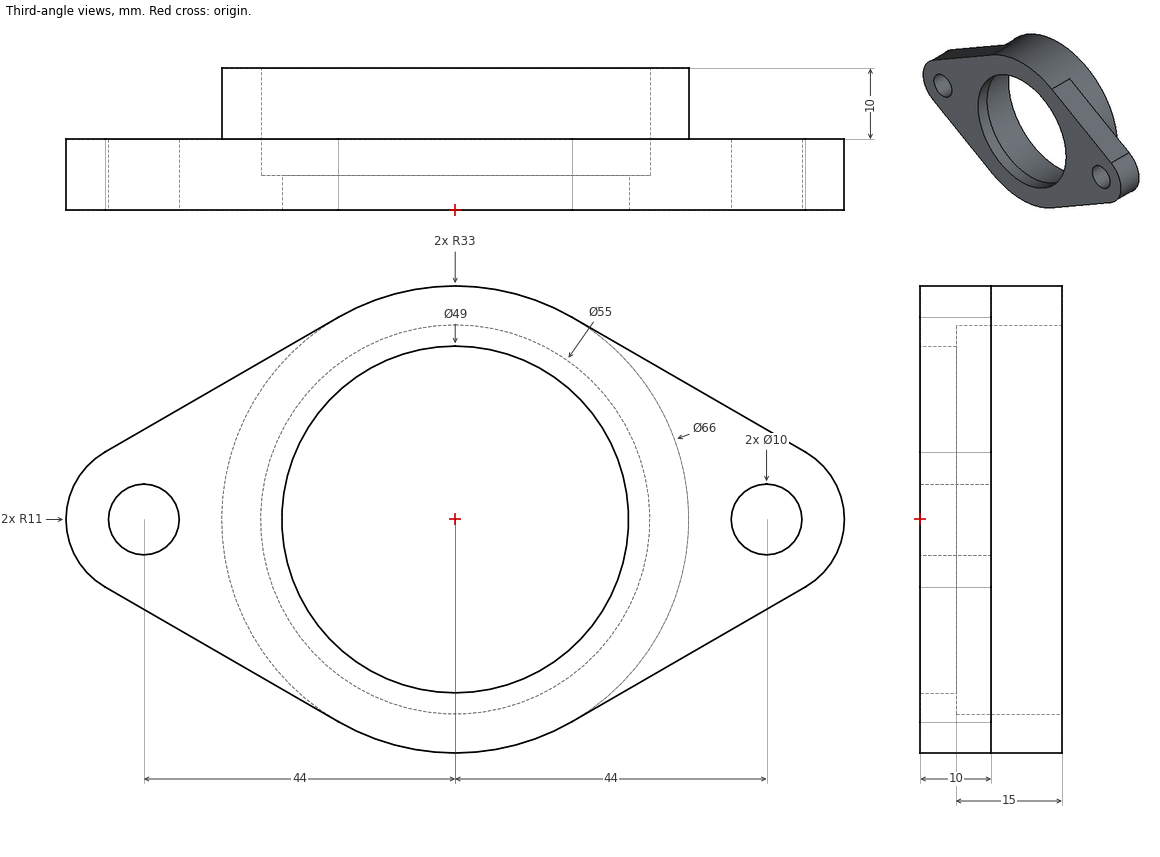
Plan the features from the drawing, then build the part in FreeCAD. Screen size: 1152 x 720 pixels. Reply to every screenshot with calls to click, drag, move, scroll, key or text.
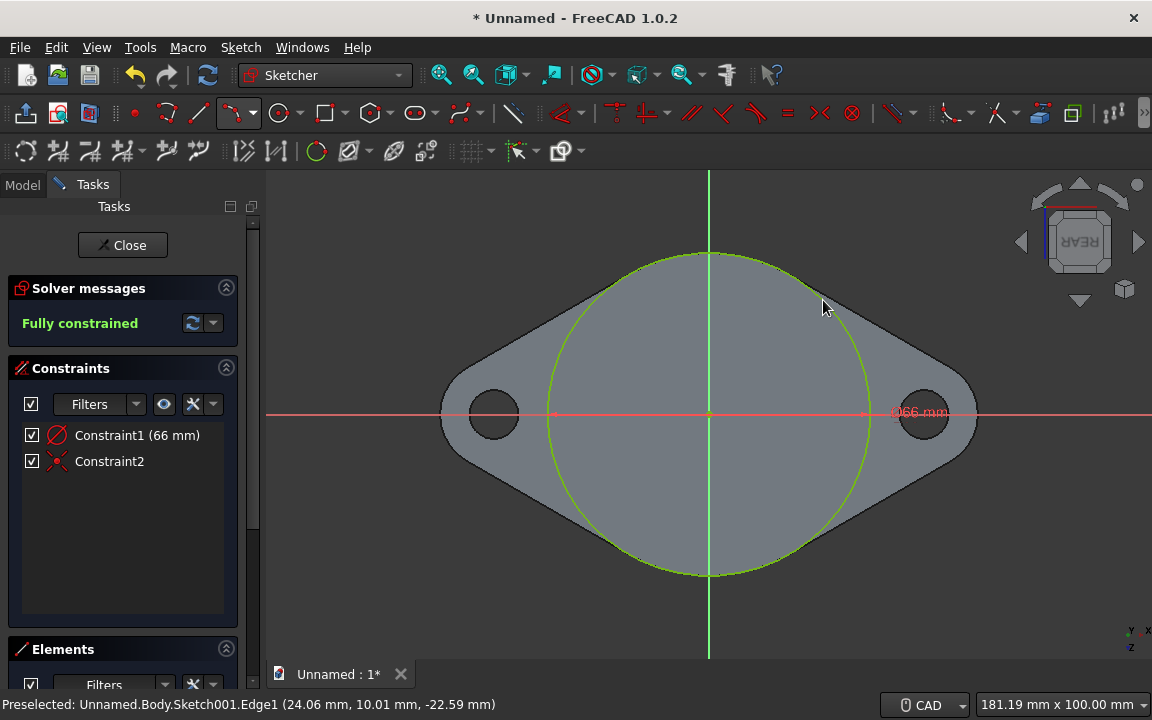
click(123, 245)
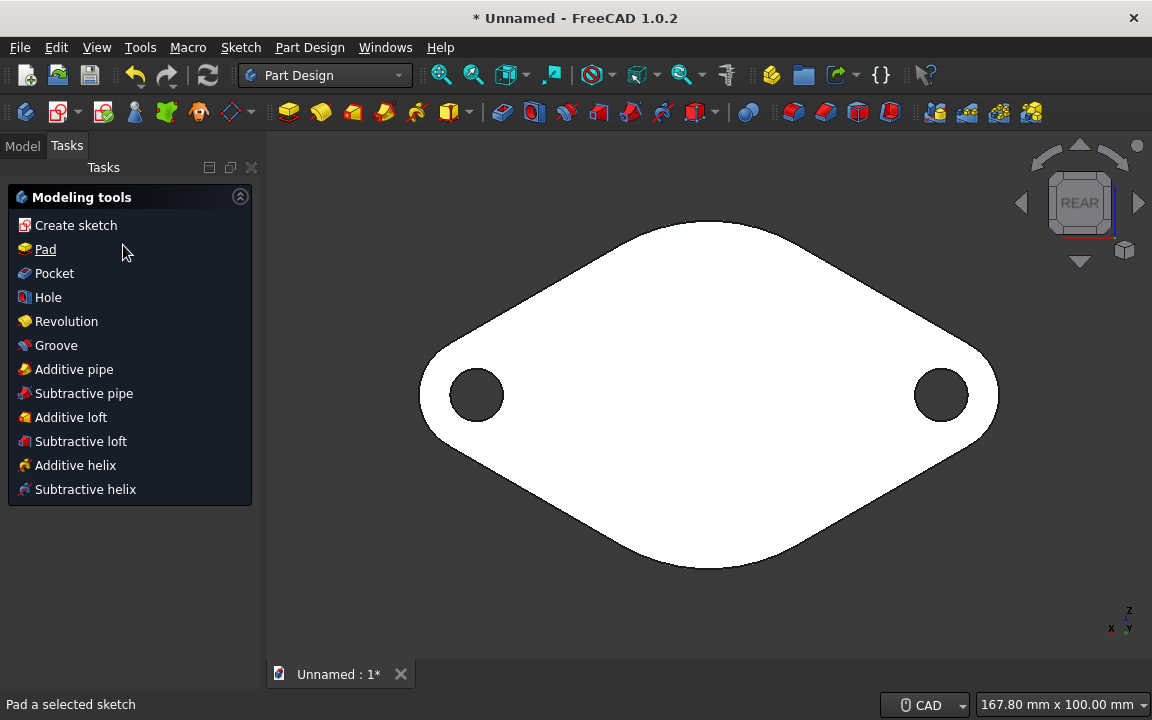
click(290, 112)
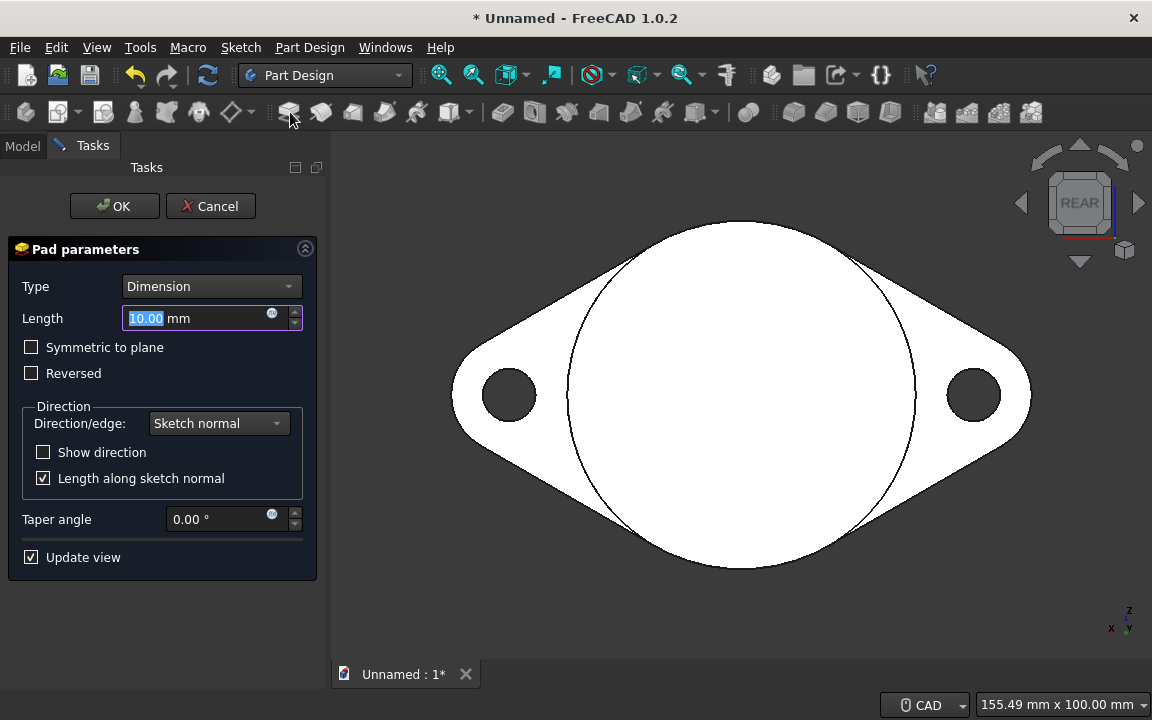
text(10)
key(Tab)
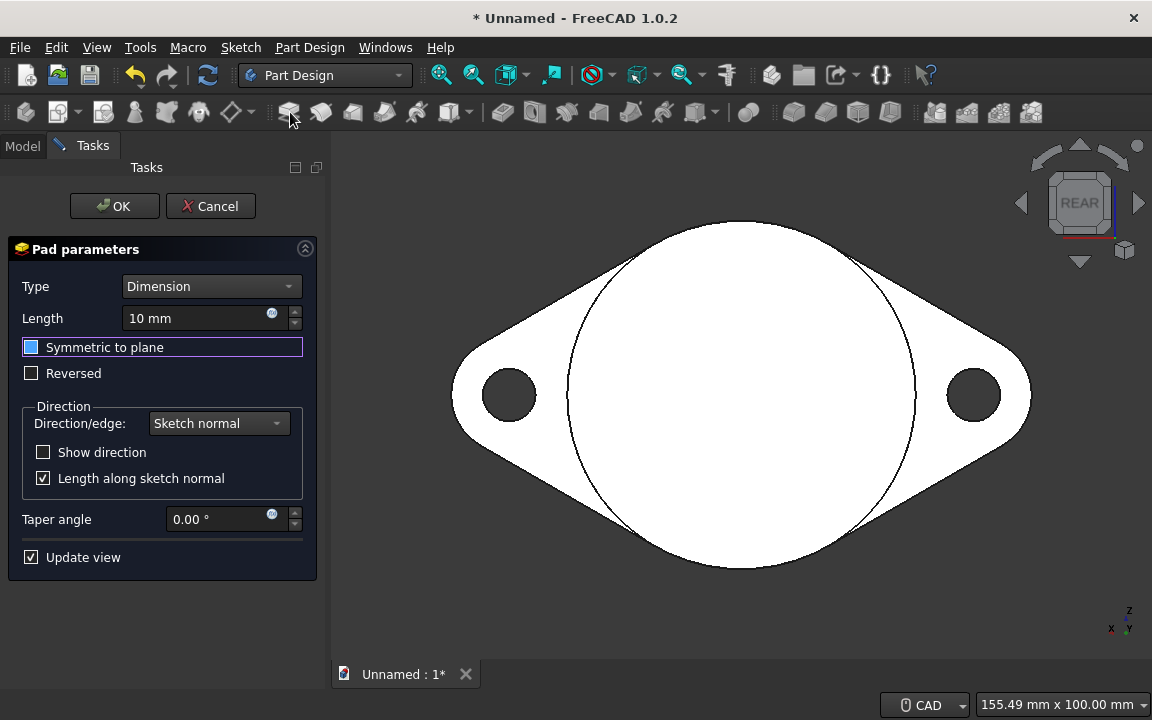
click(115, 206)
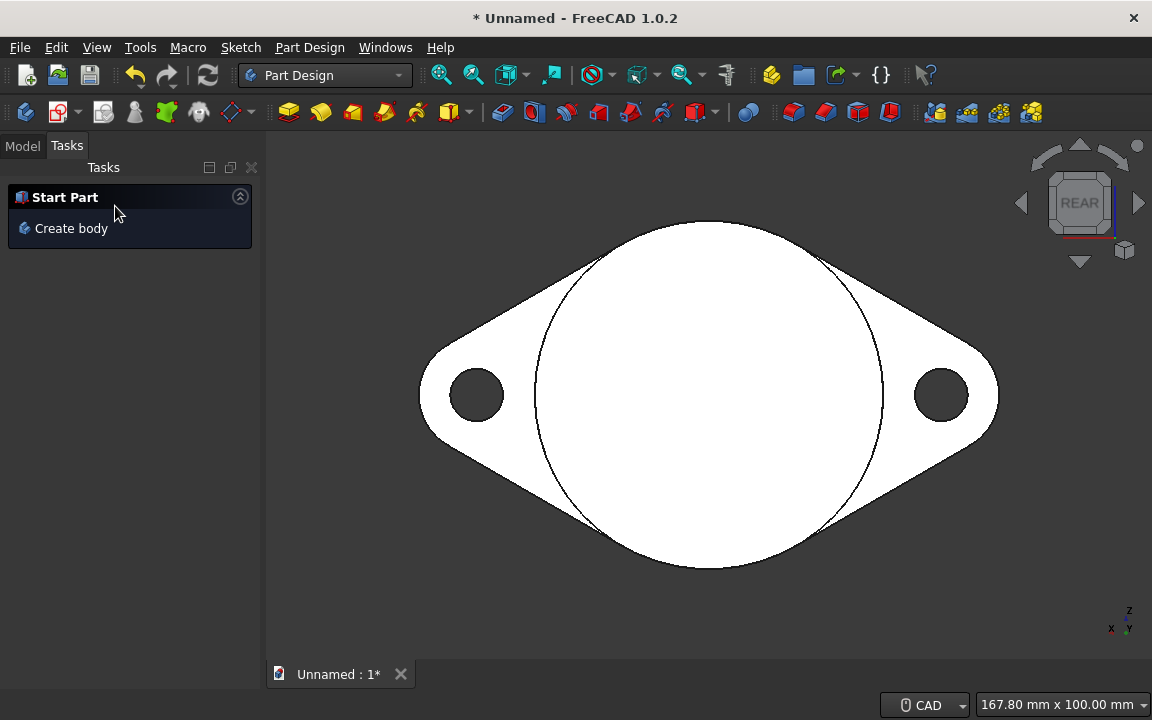
click(709, 394)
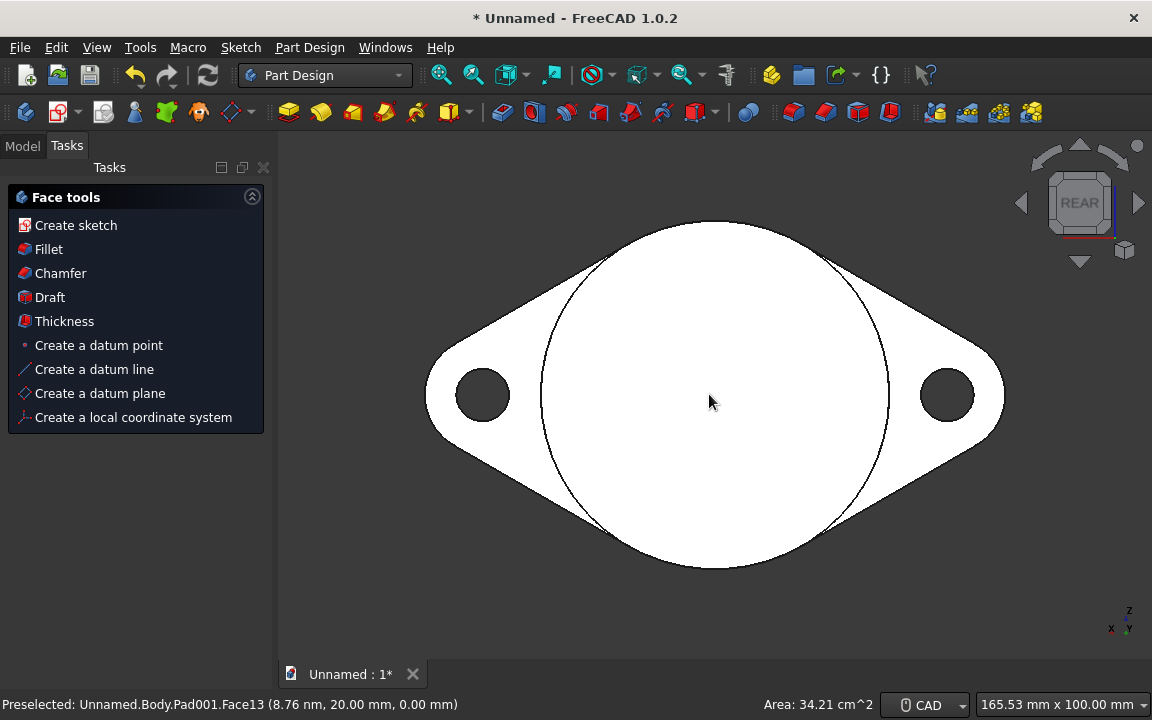
click(58, 112)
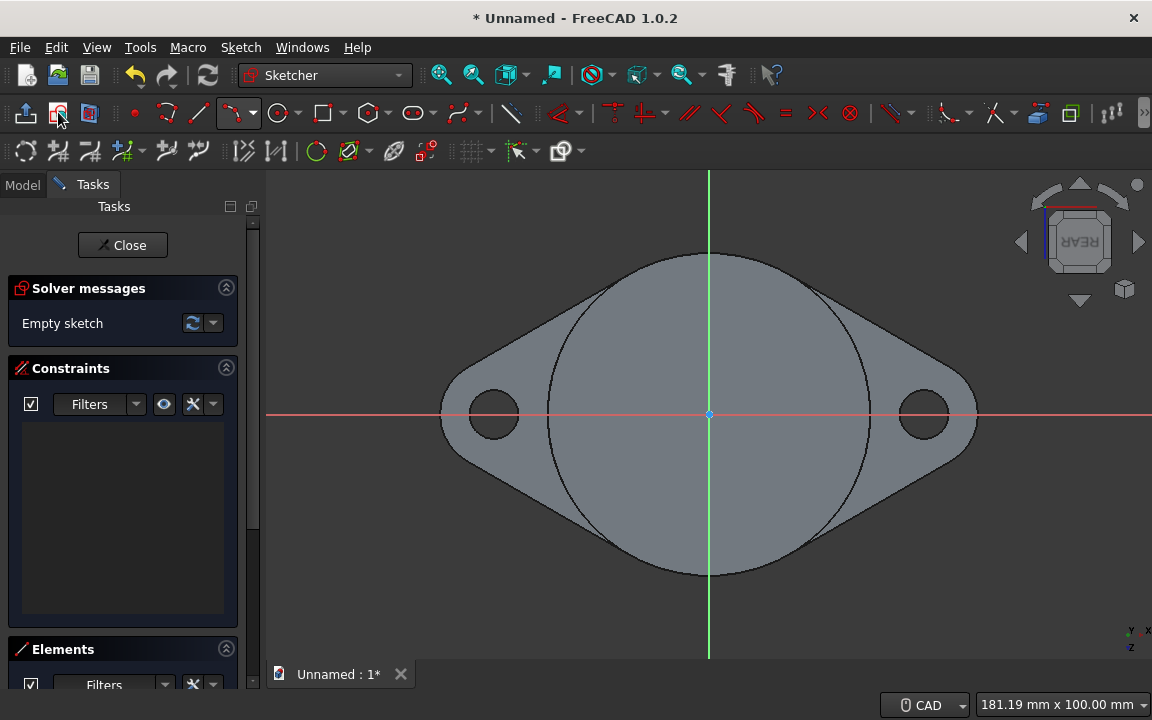
click(278, 114)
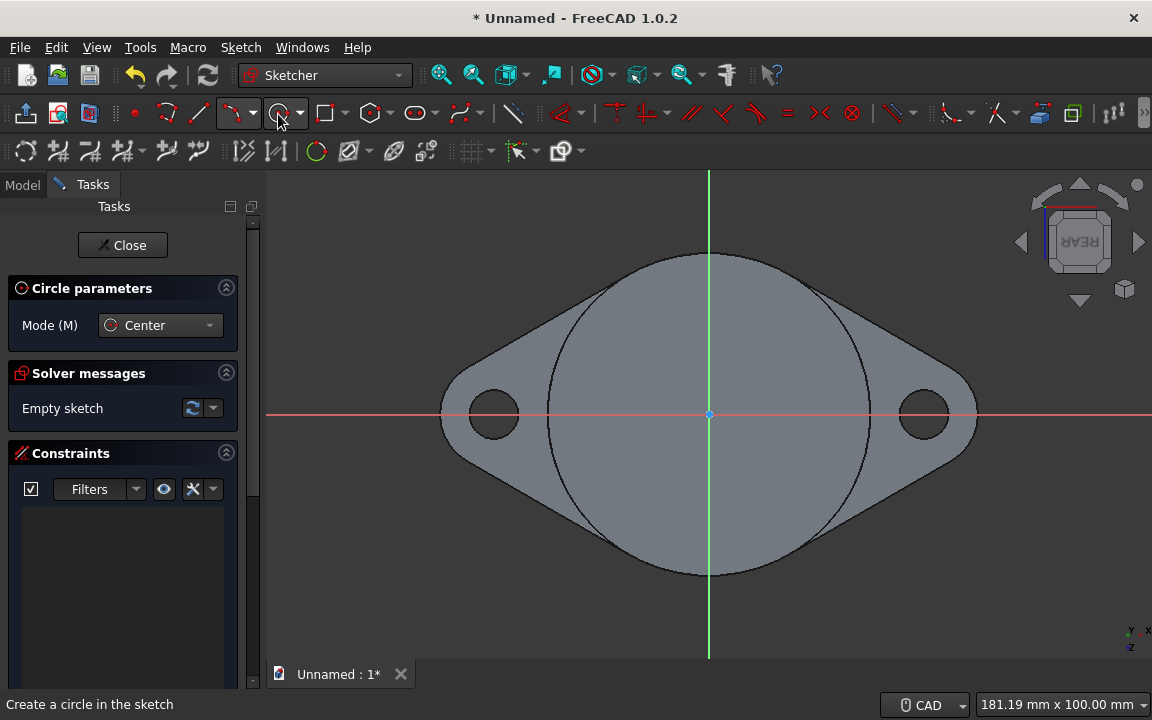
click(709, 414)
move(804, 319)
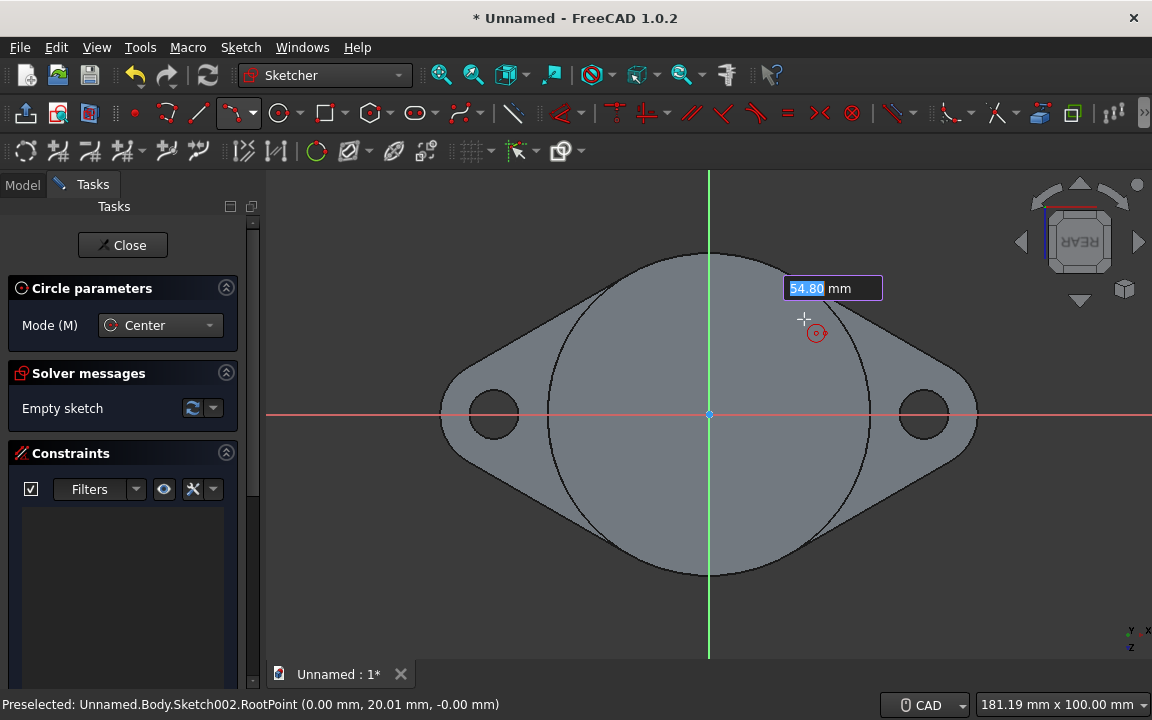
text(55)
key(Return)
key(Escape)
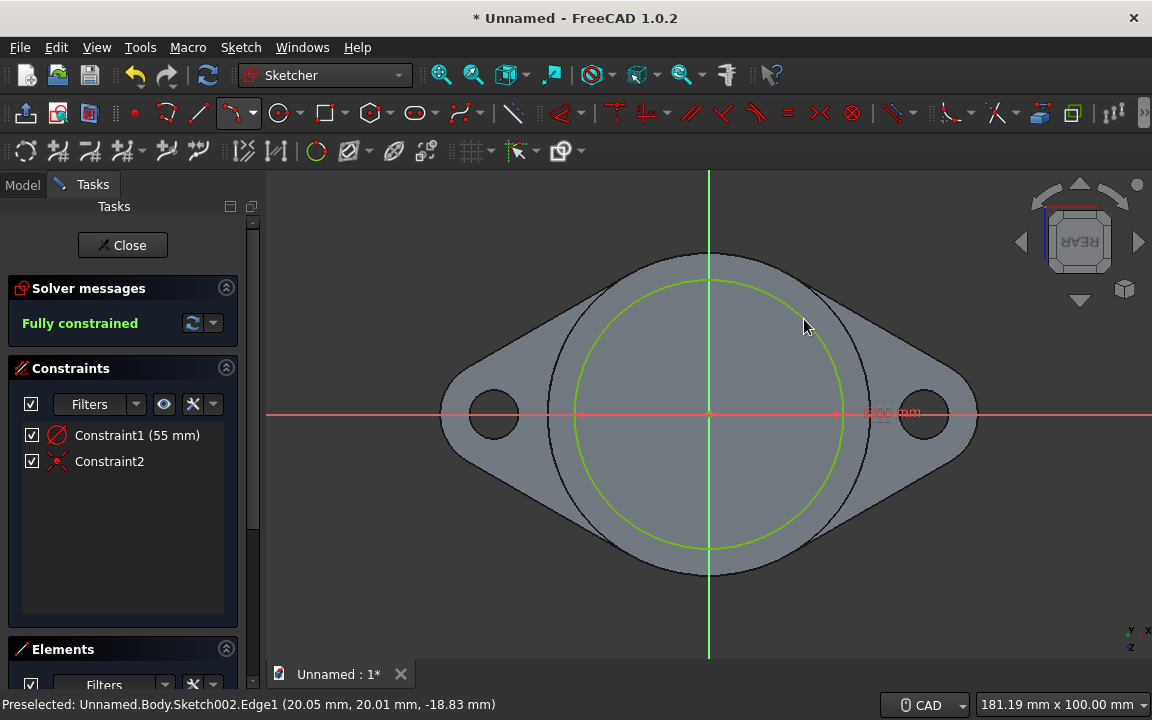
click(123, 245)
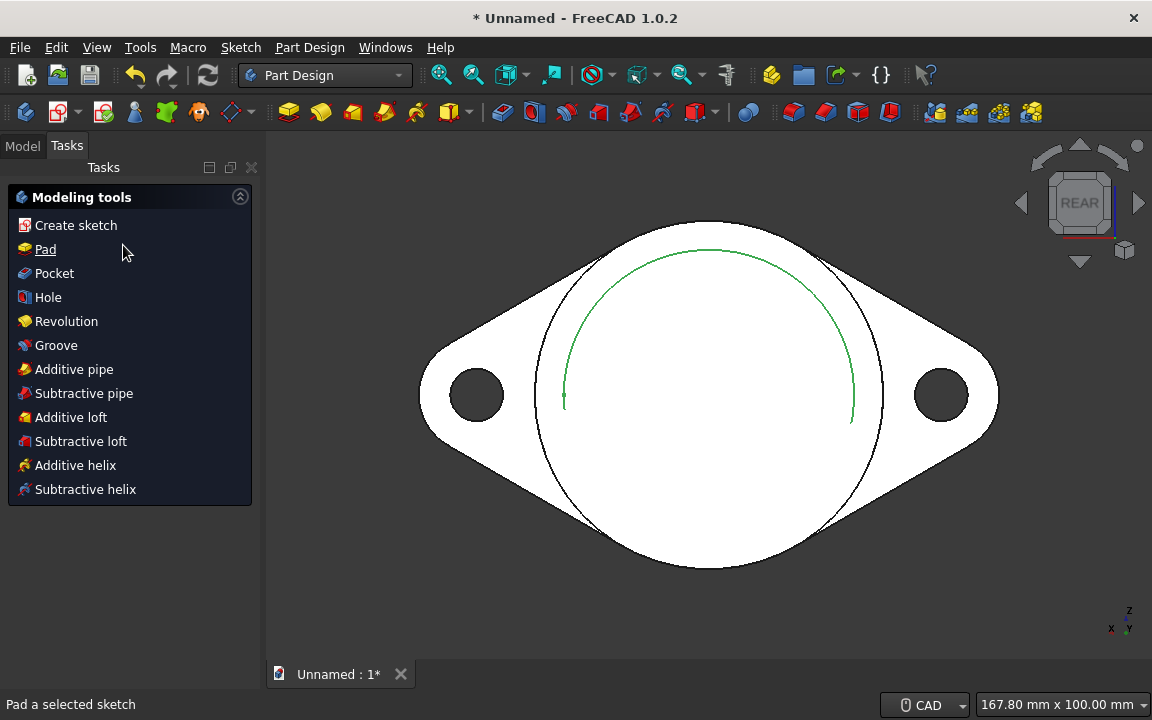
click(504, 112)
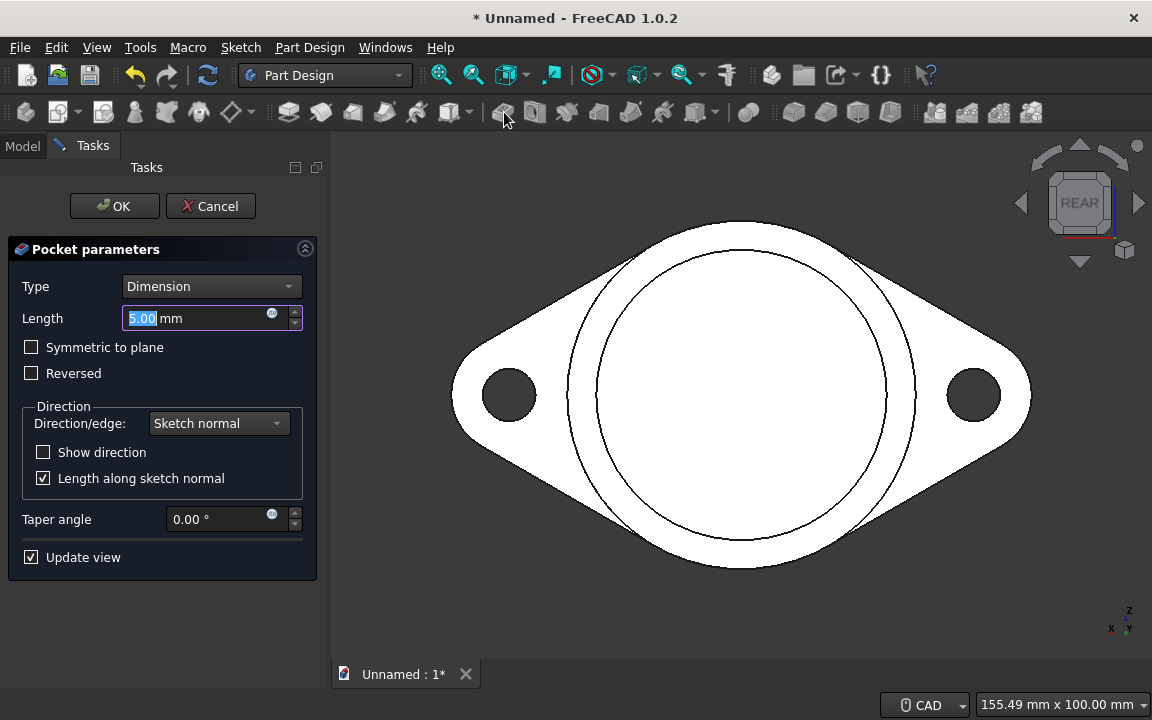
text(15)
key(Tab)